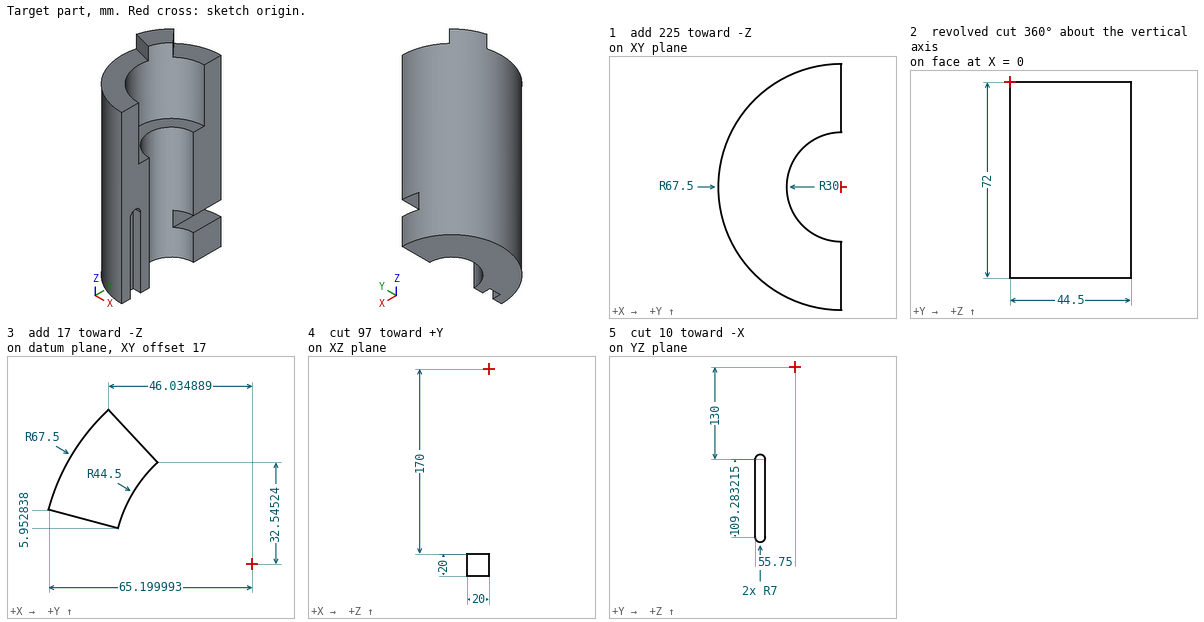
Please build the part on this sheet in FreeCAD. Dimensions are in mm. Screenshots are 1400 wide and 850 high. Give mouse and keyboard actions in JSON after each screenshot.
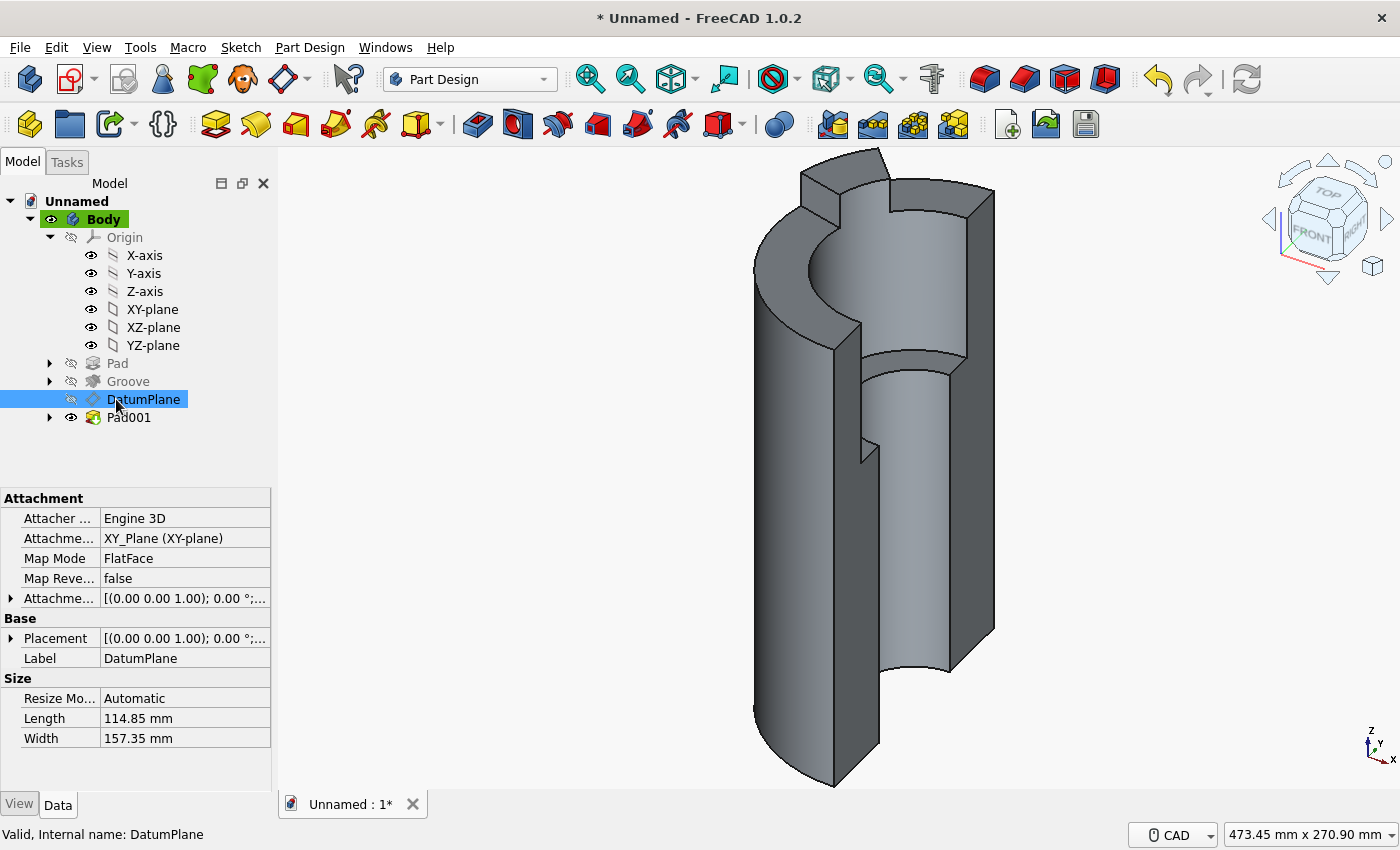
{"action": "key", "text": "v f"}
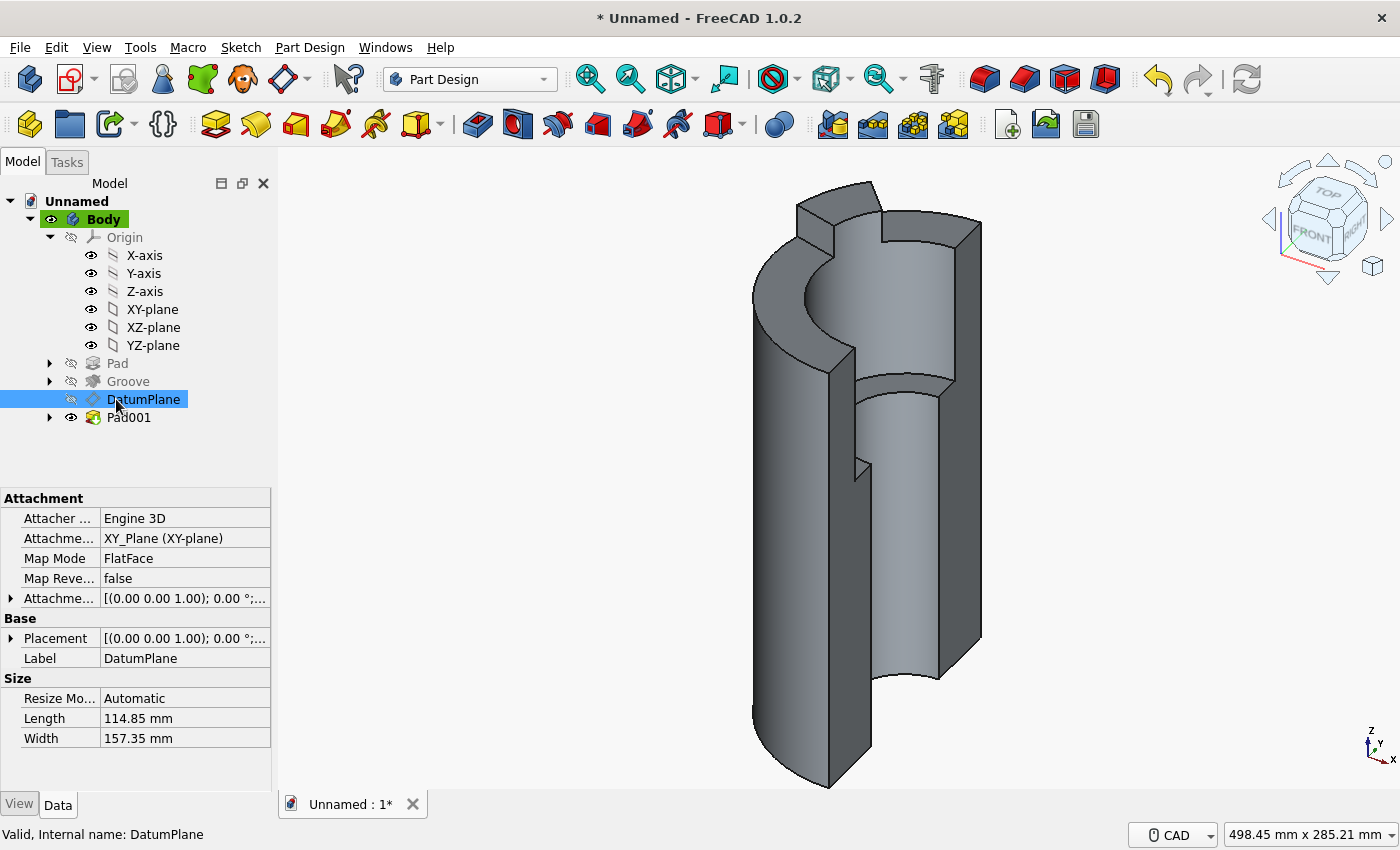
{"action": "left_click", "coordinate": [318, 749]}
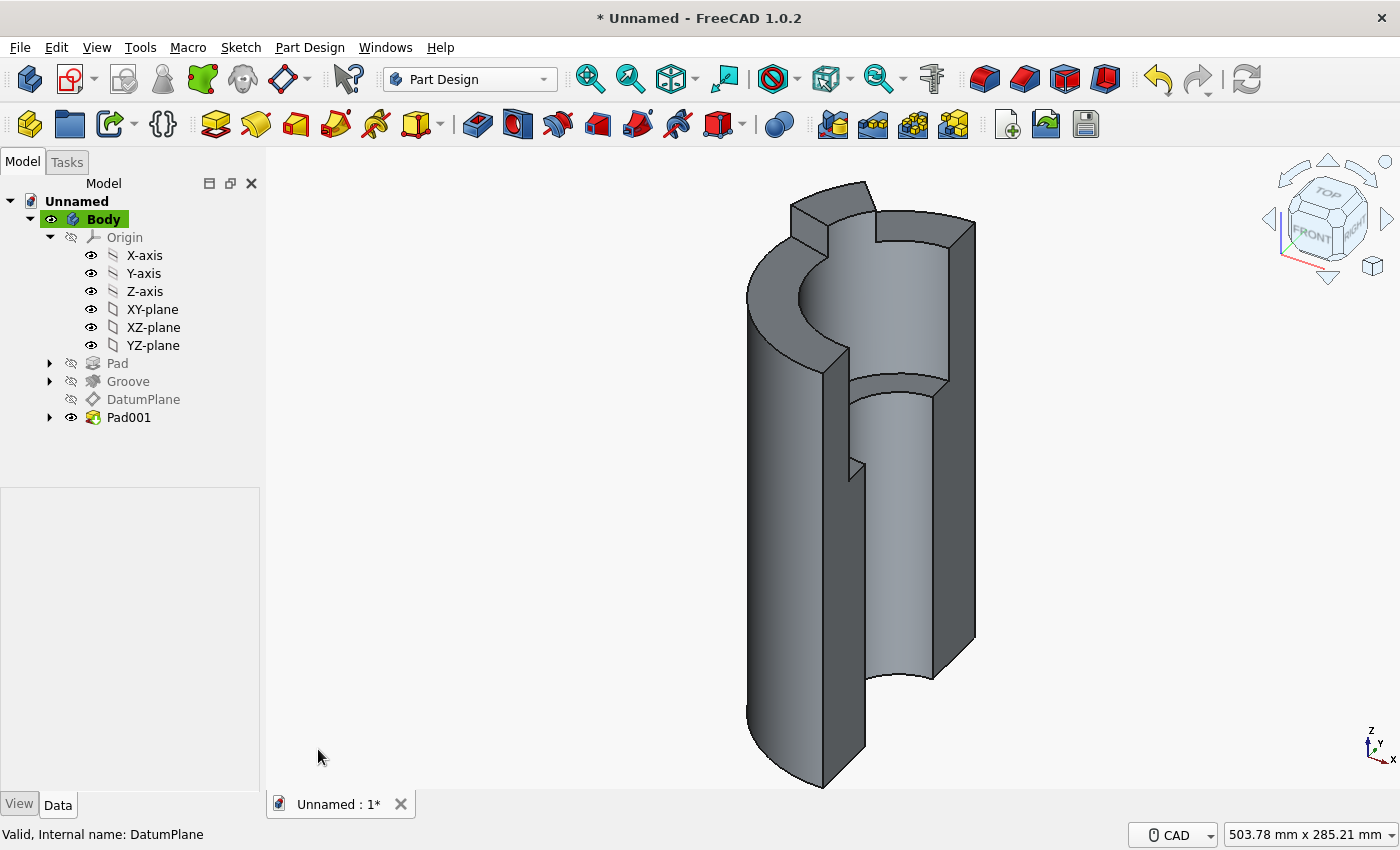
{"action": "left_click", "coordinate": [70, 80]}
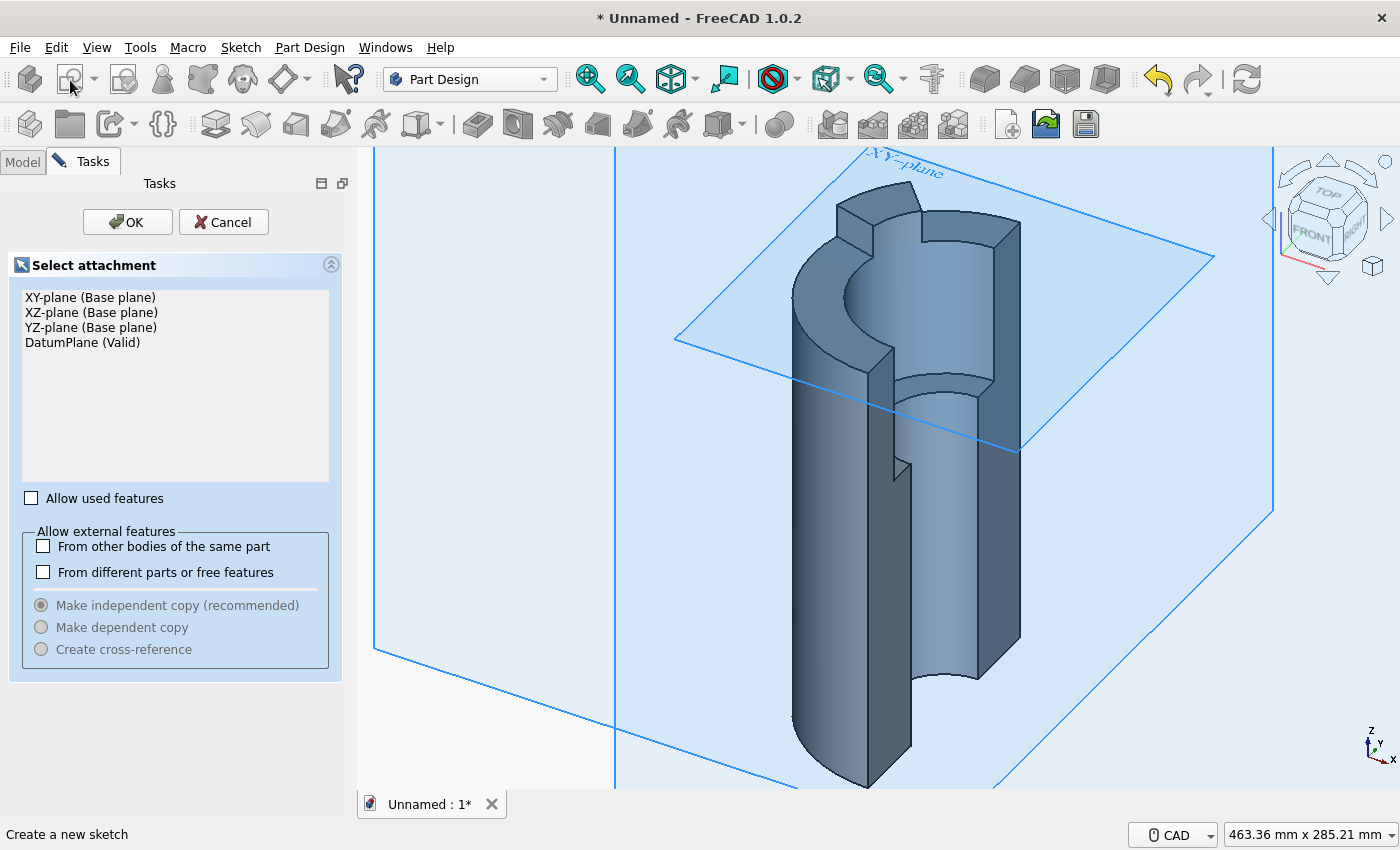
{"action": "left_click", "coordinate": [82, 312]}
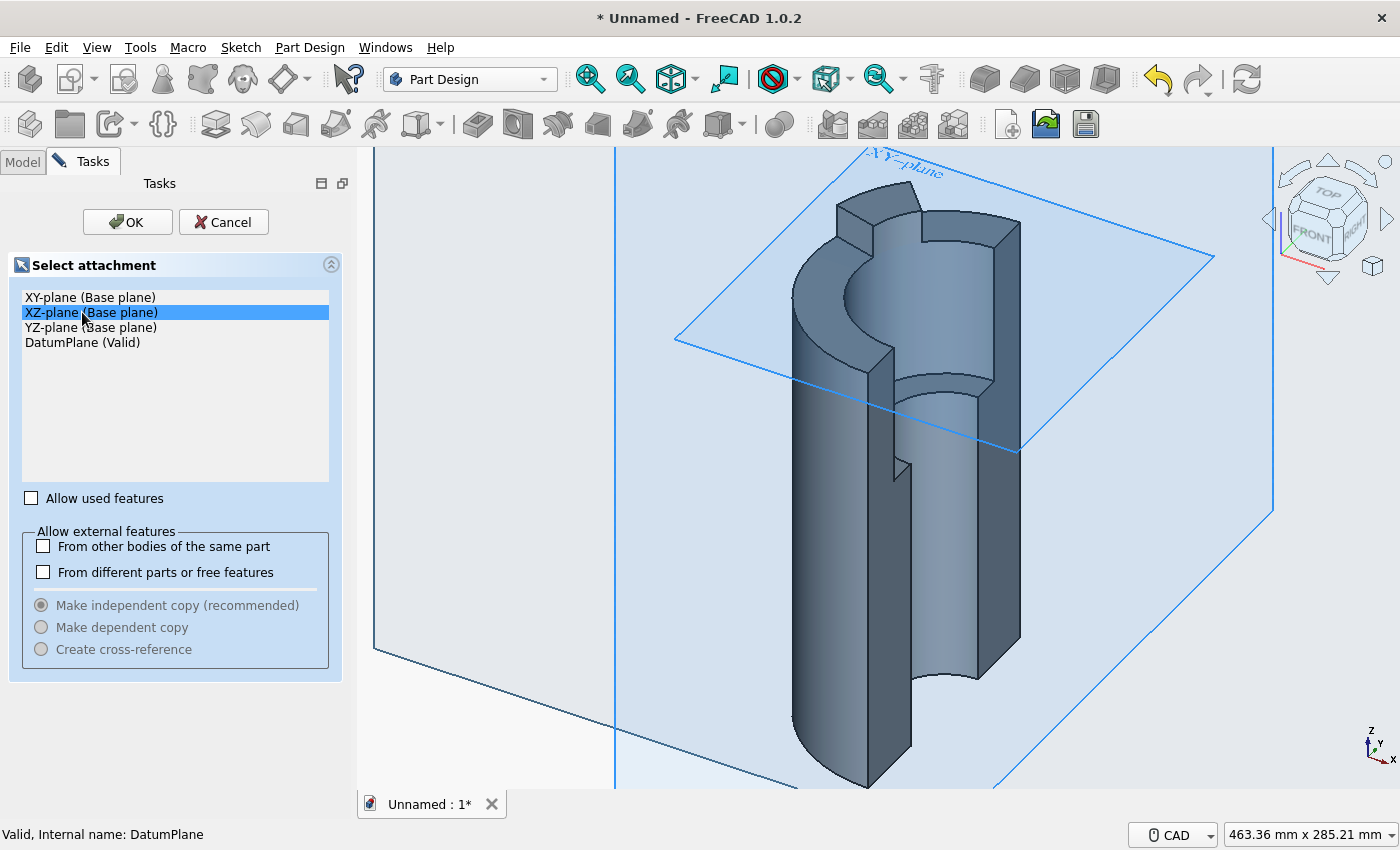
{"action": "left_click", "coordinate": [128, 222]}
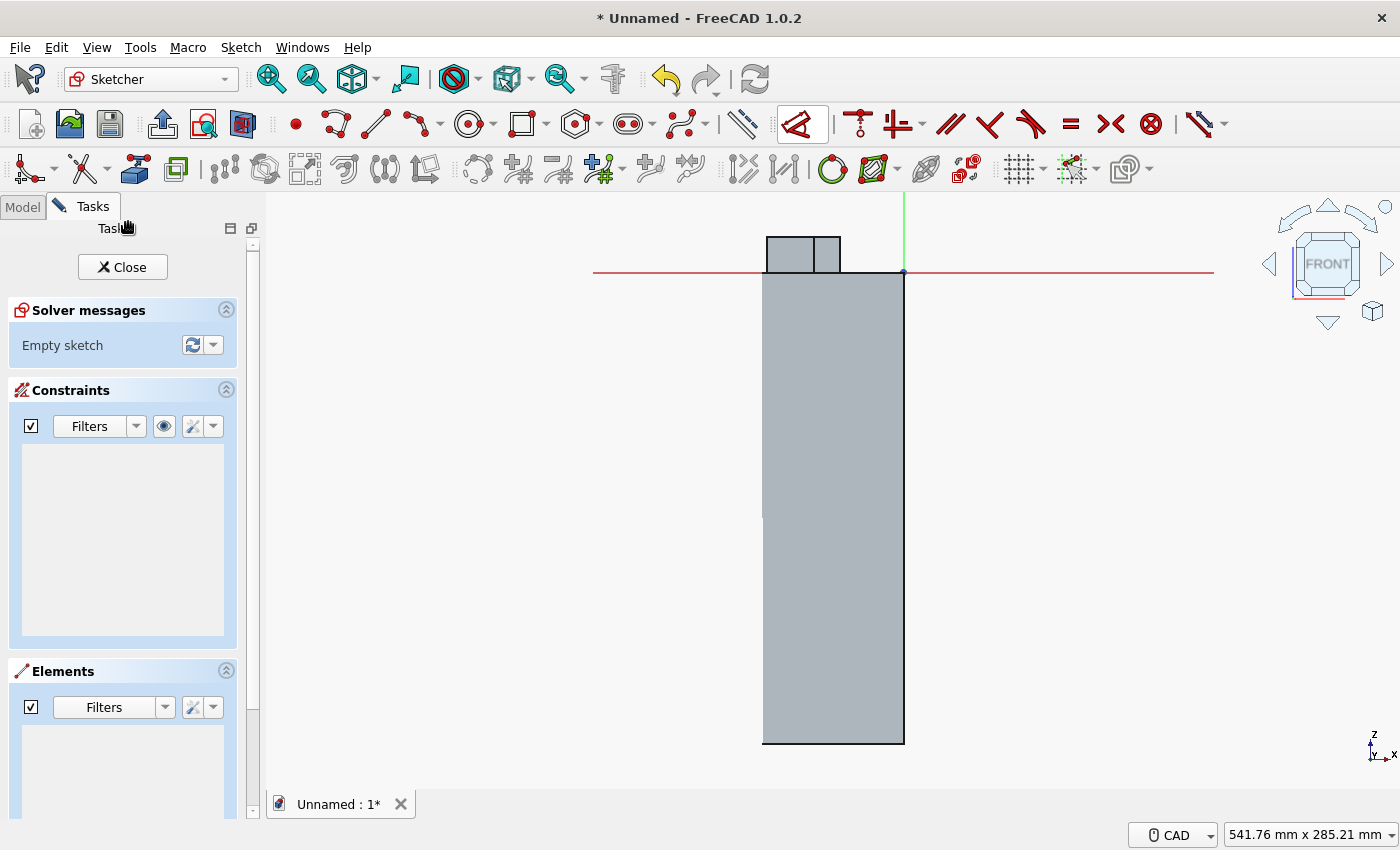
{"action": "key", "text": "q s"}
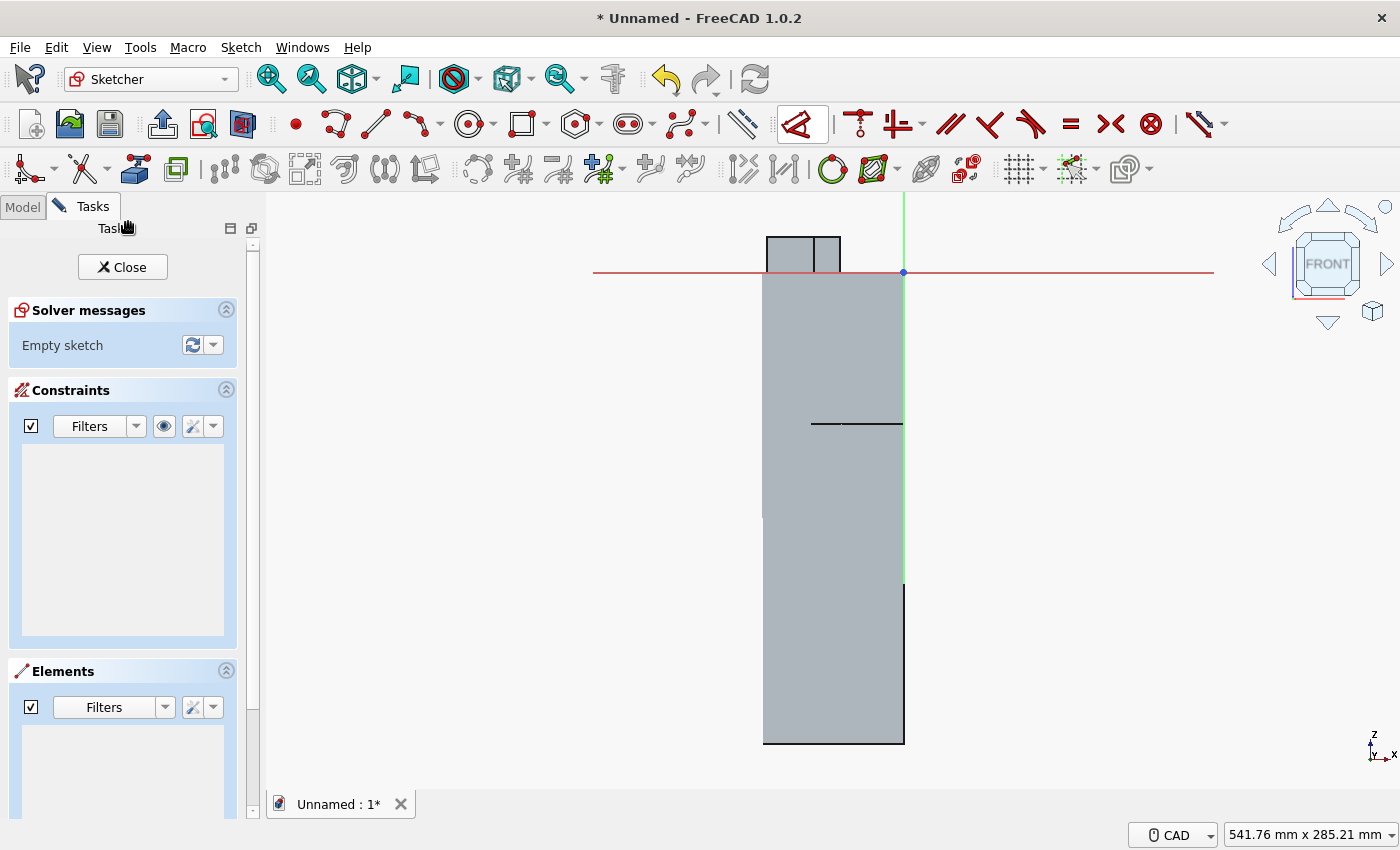
{"action": "scroll", "coordinate": [897, 669], "scroll_direction": "up", "scroll_amount": 11}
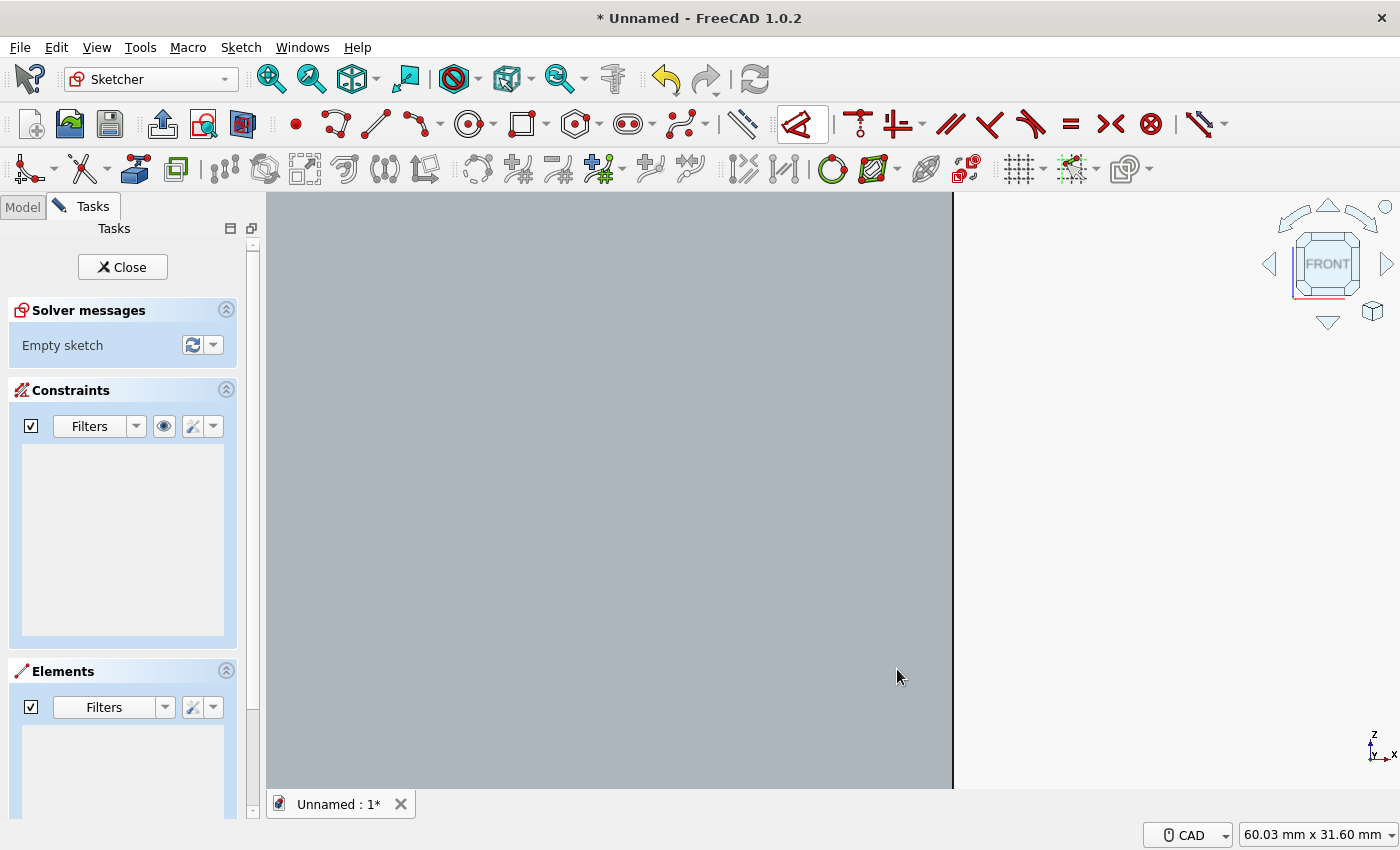
{"action": "left_click", "coordinate": [522, 124]}